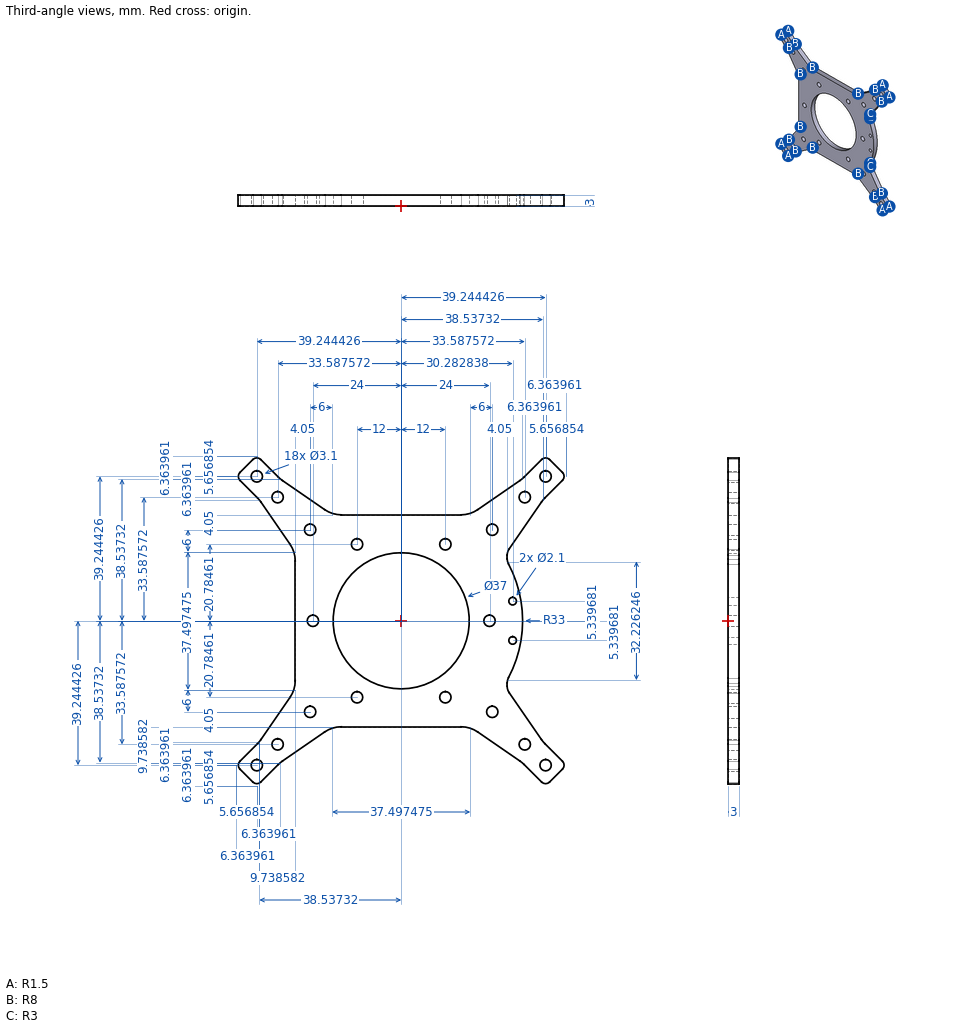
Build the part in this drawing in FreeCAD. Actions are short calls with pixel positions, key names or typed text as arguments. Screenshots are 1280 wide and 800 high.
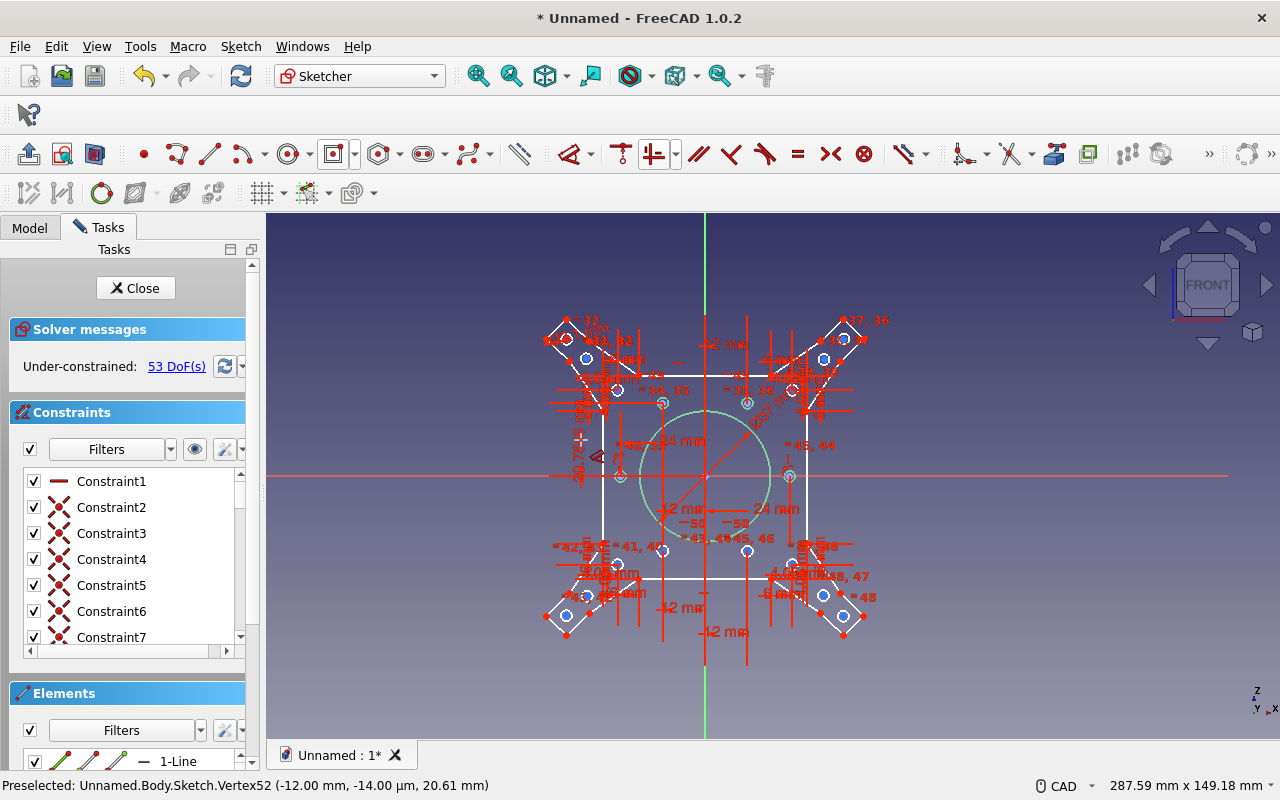
click(663, 551)
click(629, 531)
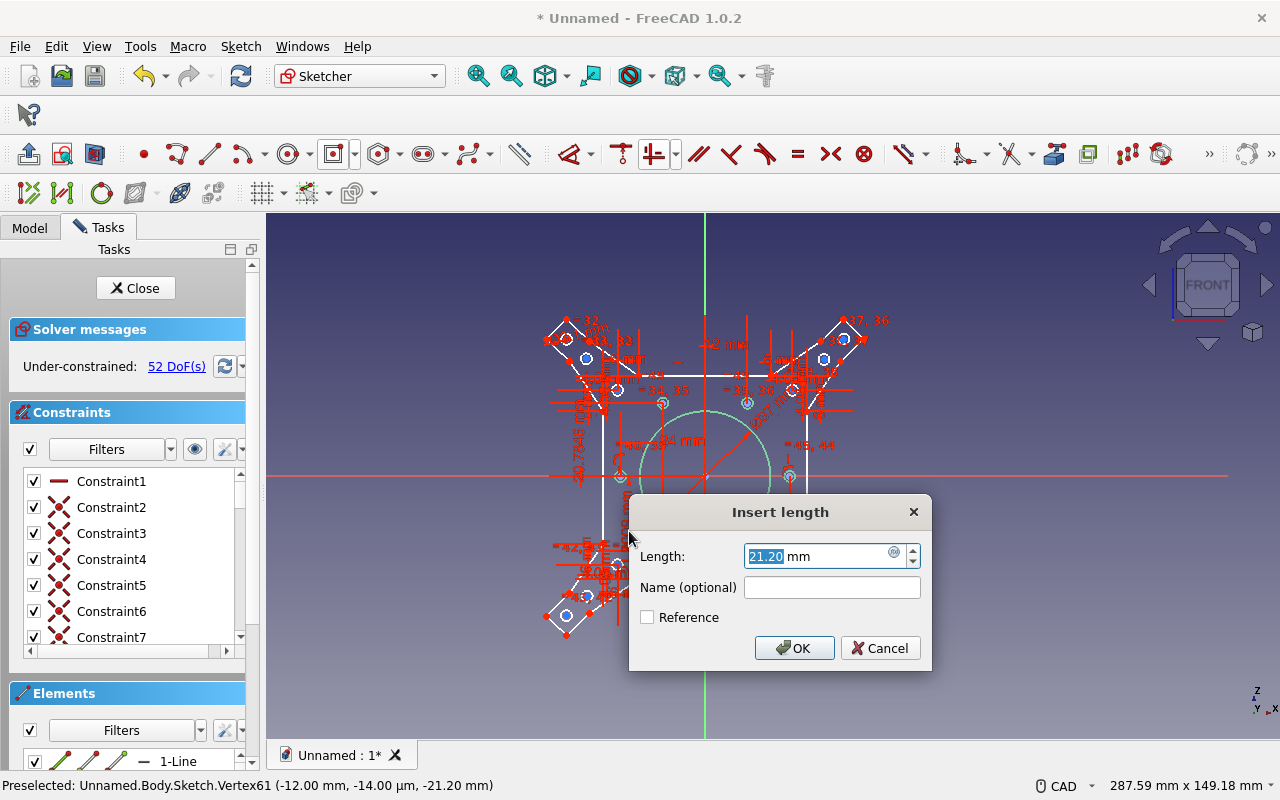
text(20.78461)
key(Return)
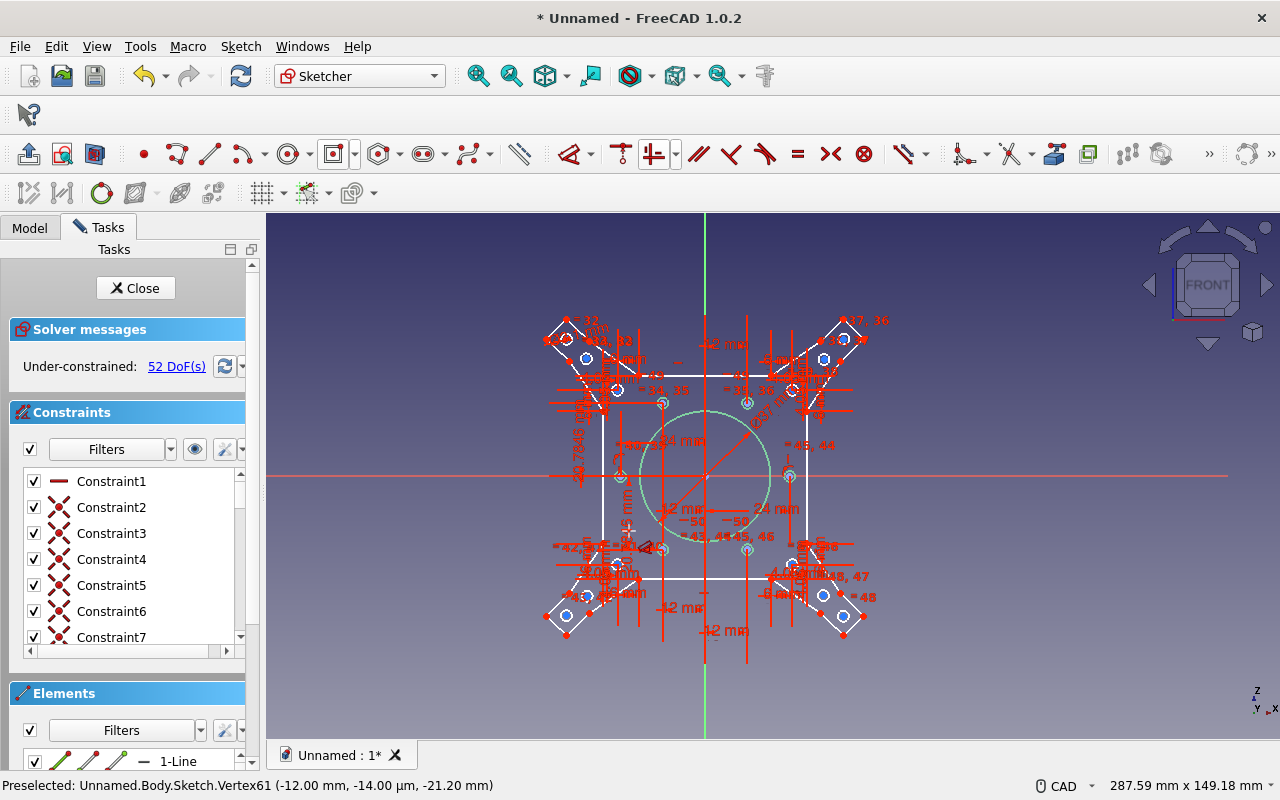
click(732, 579)
click(674, 661)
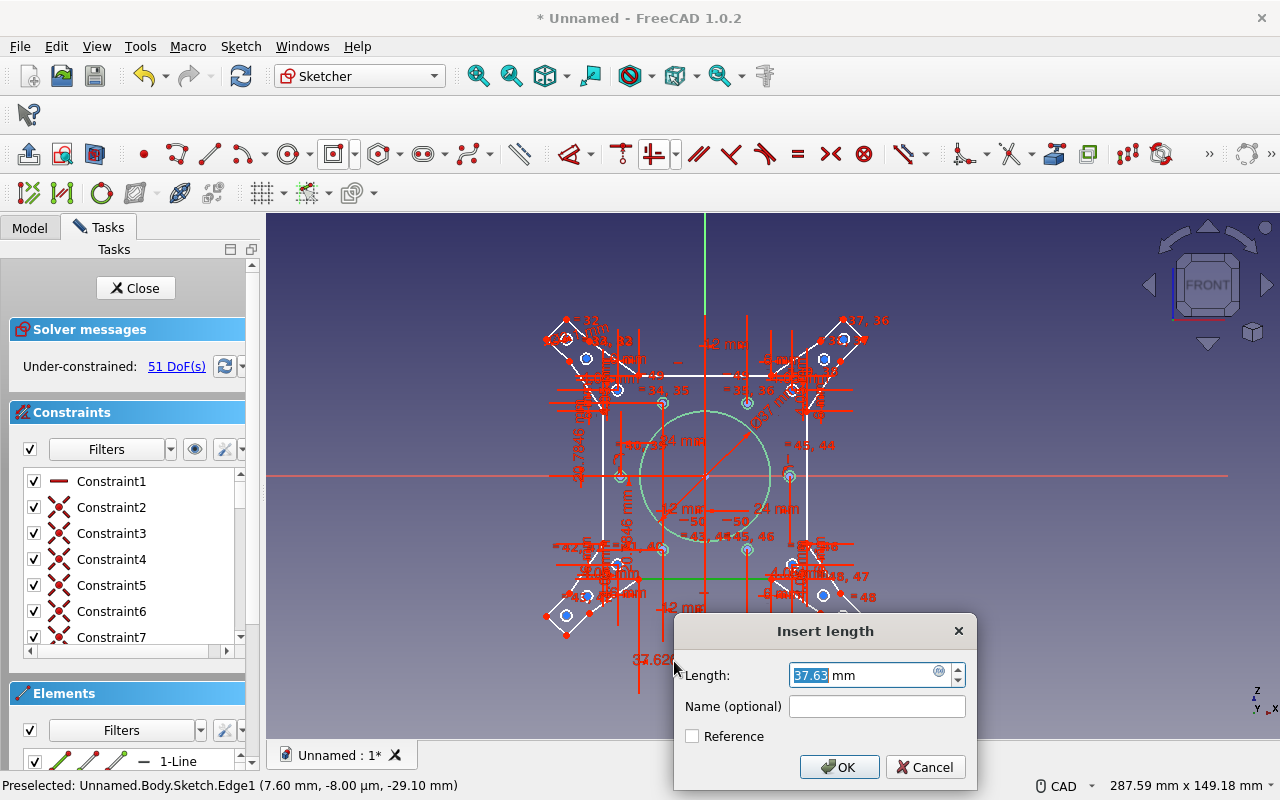
text(37.497475)
key(Return)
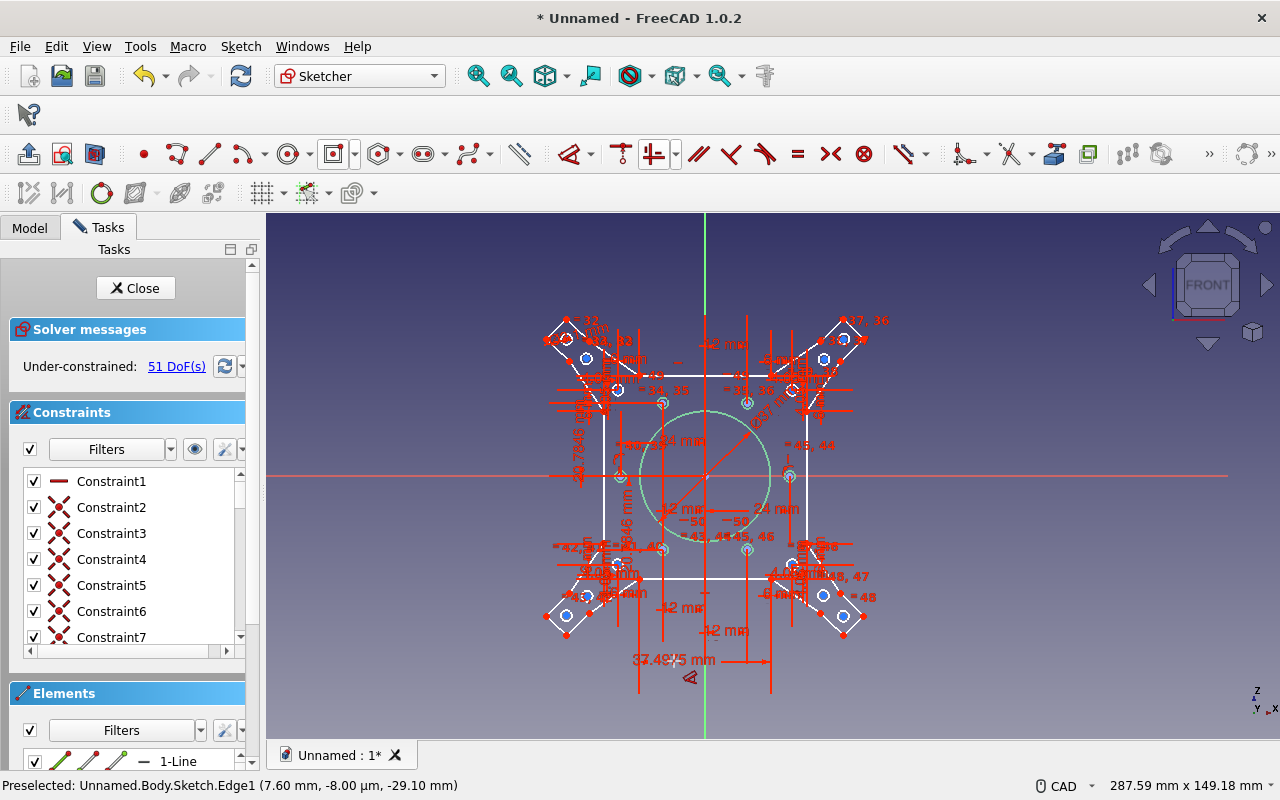
click(604, 504)
click(570, 508)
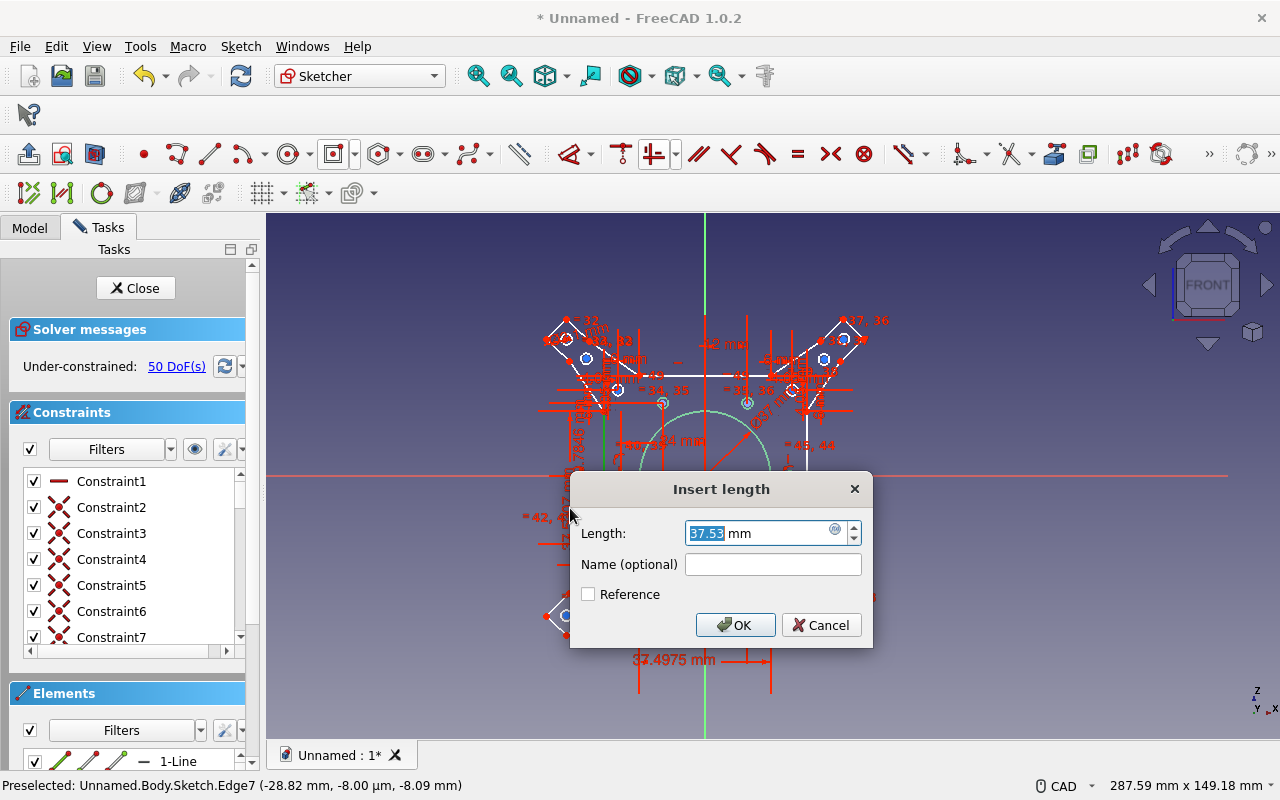
text(37.497475)
key(Return)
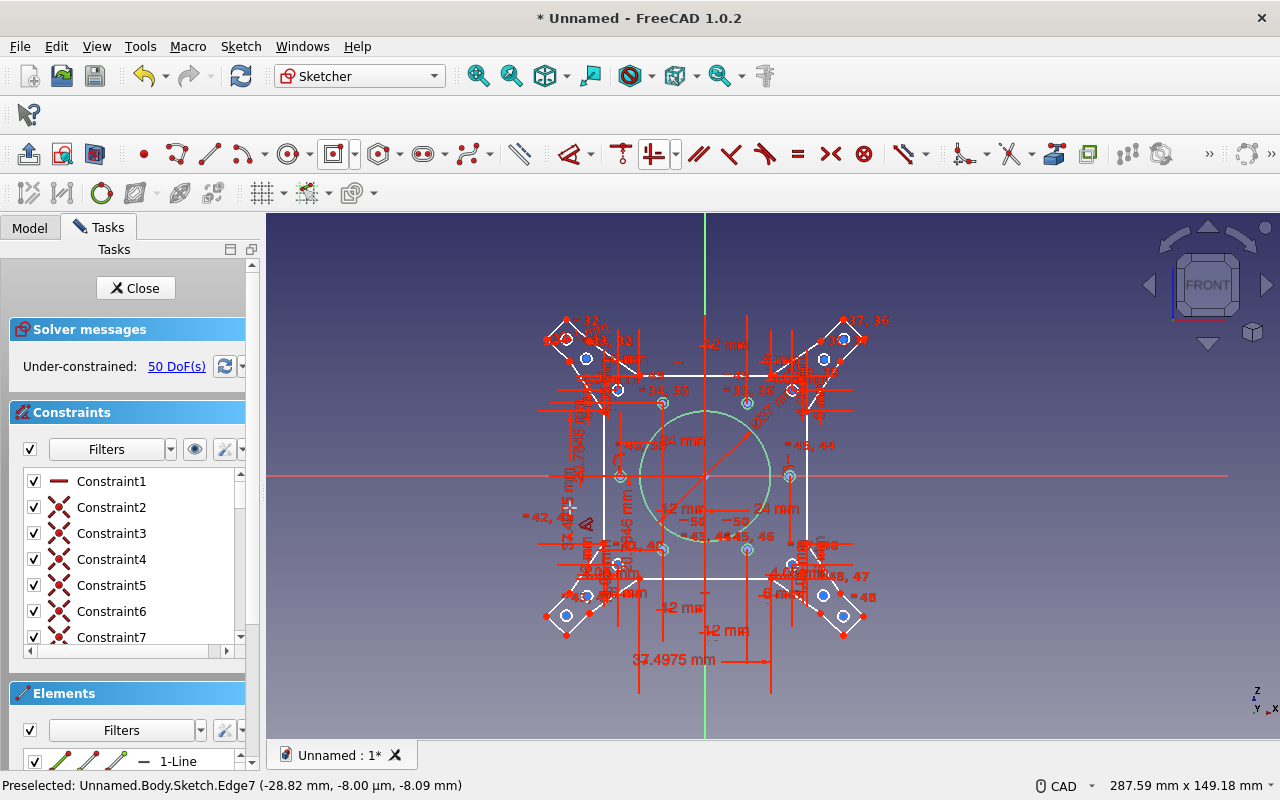
click(590, 613)
click(532, 576)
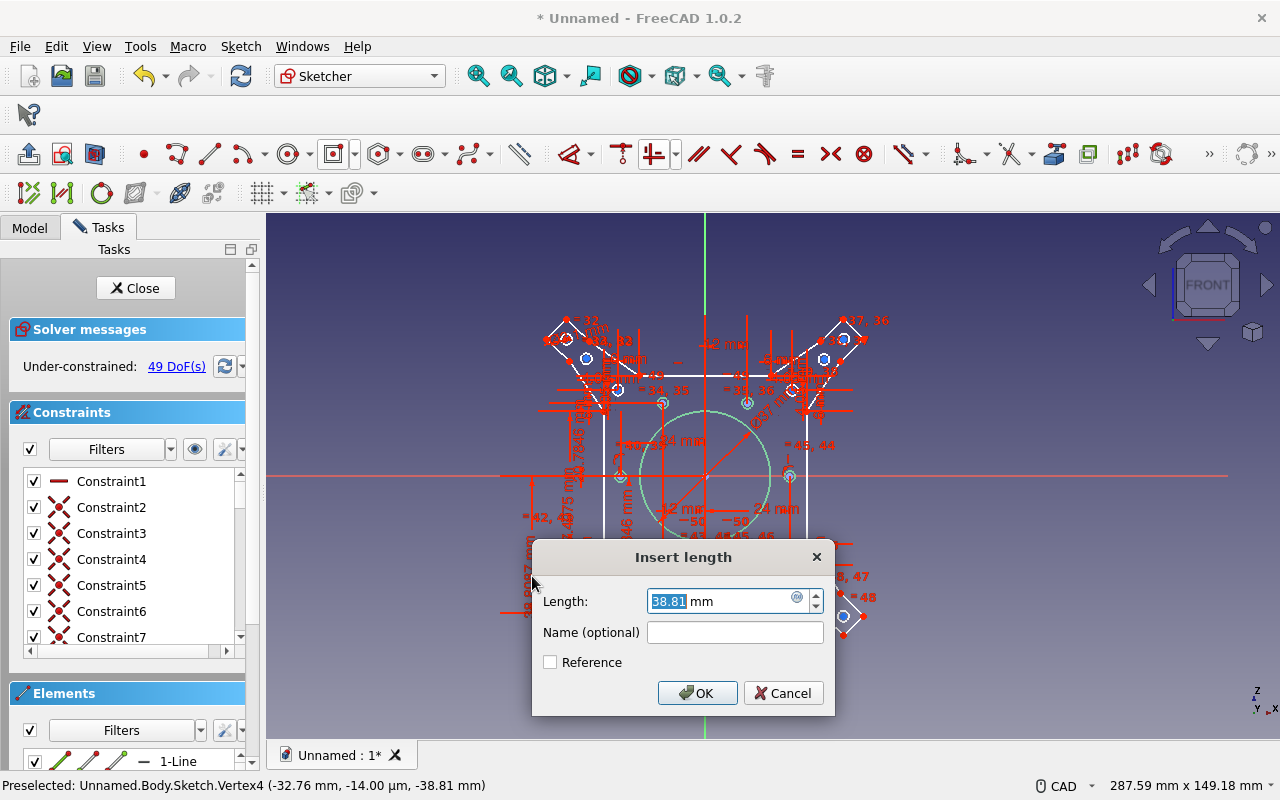
text(38.53732)
key(Return)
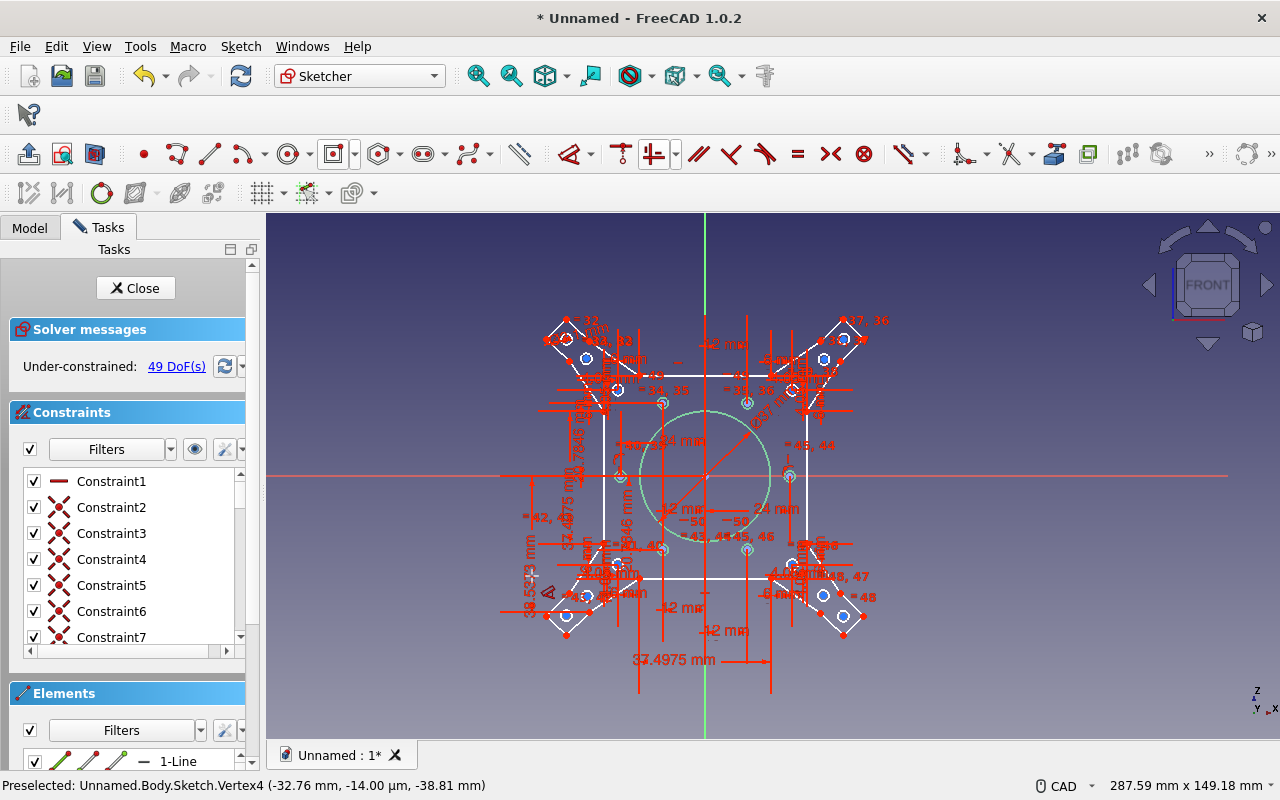
click(570, 593)
click(606, 627)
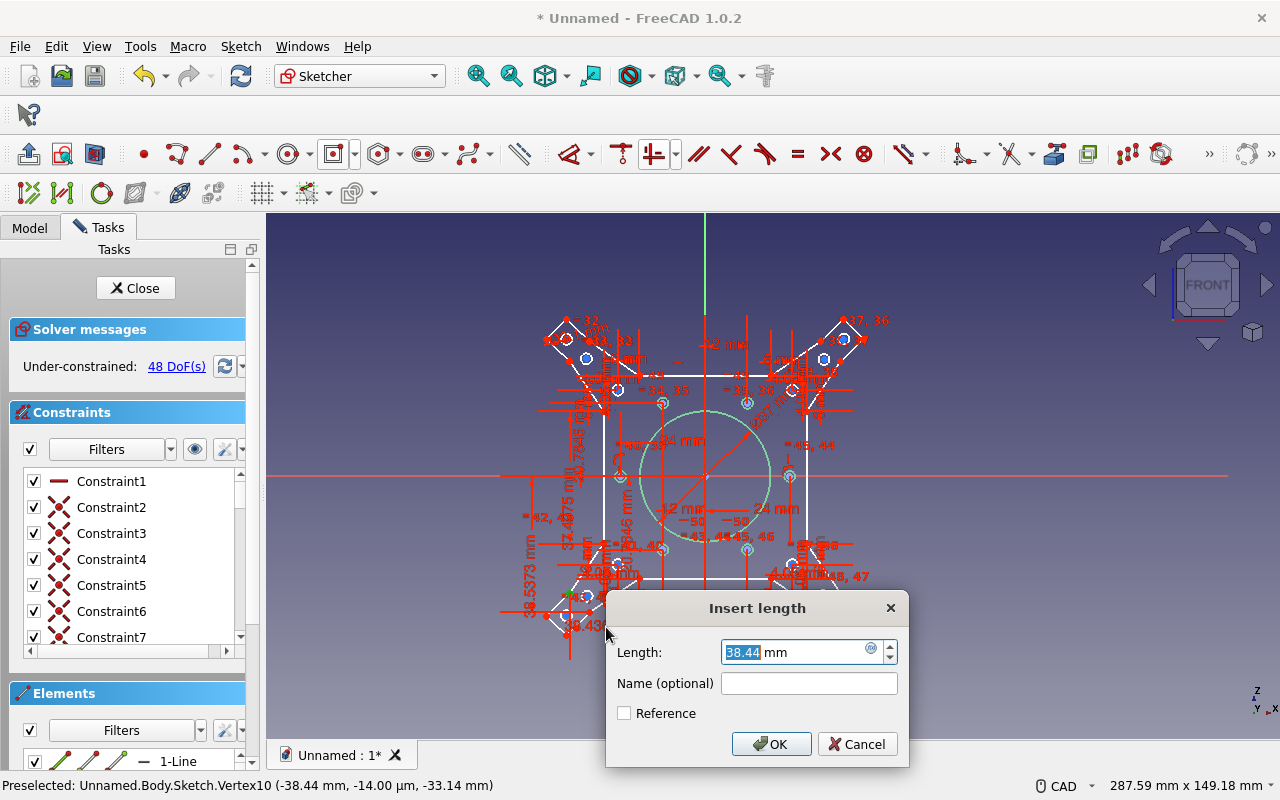
text(38.53732)
key(Return)